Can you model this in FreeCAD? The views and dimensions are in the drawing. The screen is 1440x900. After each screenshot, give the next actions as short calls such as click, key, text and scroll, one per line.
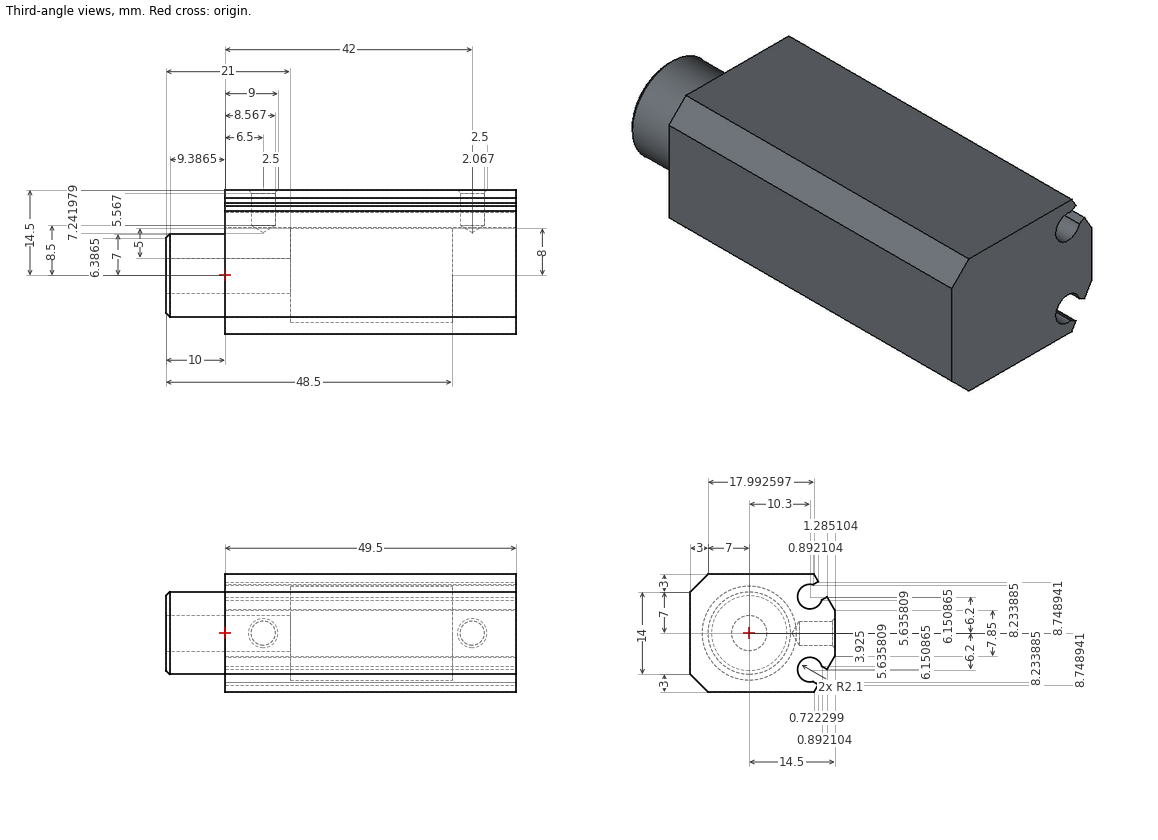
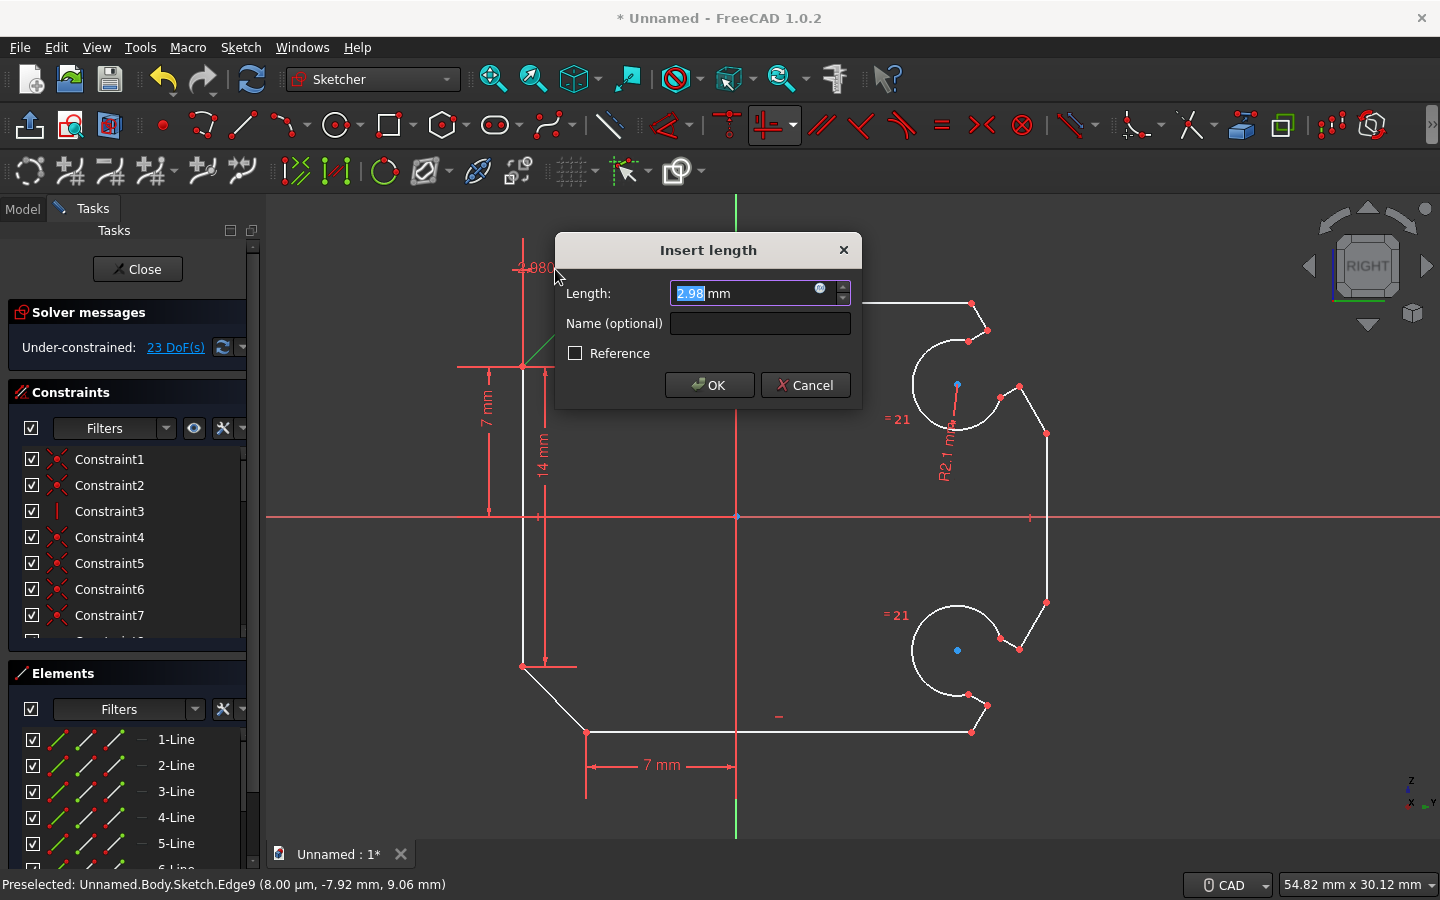
text(3)
key(Return)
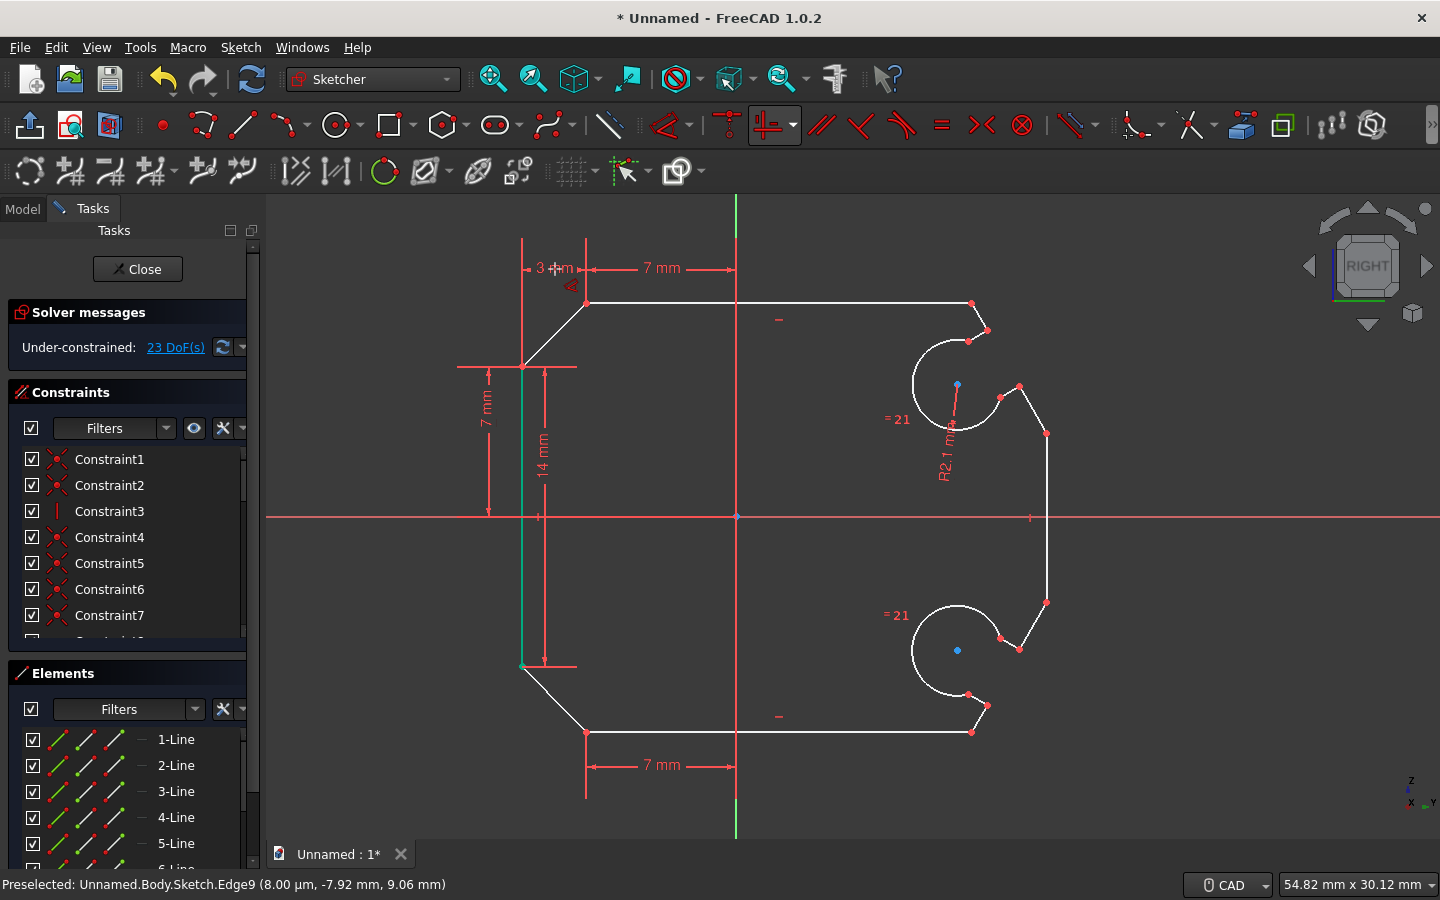
click(567, 322)
click(488, 335)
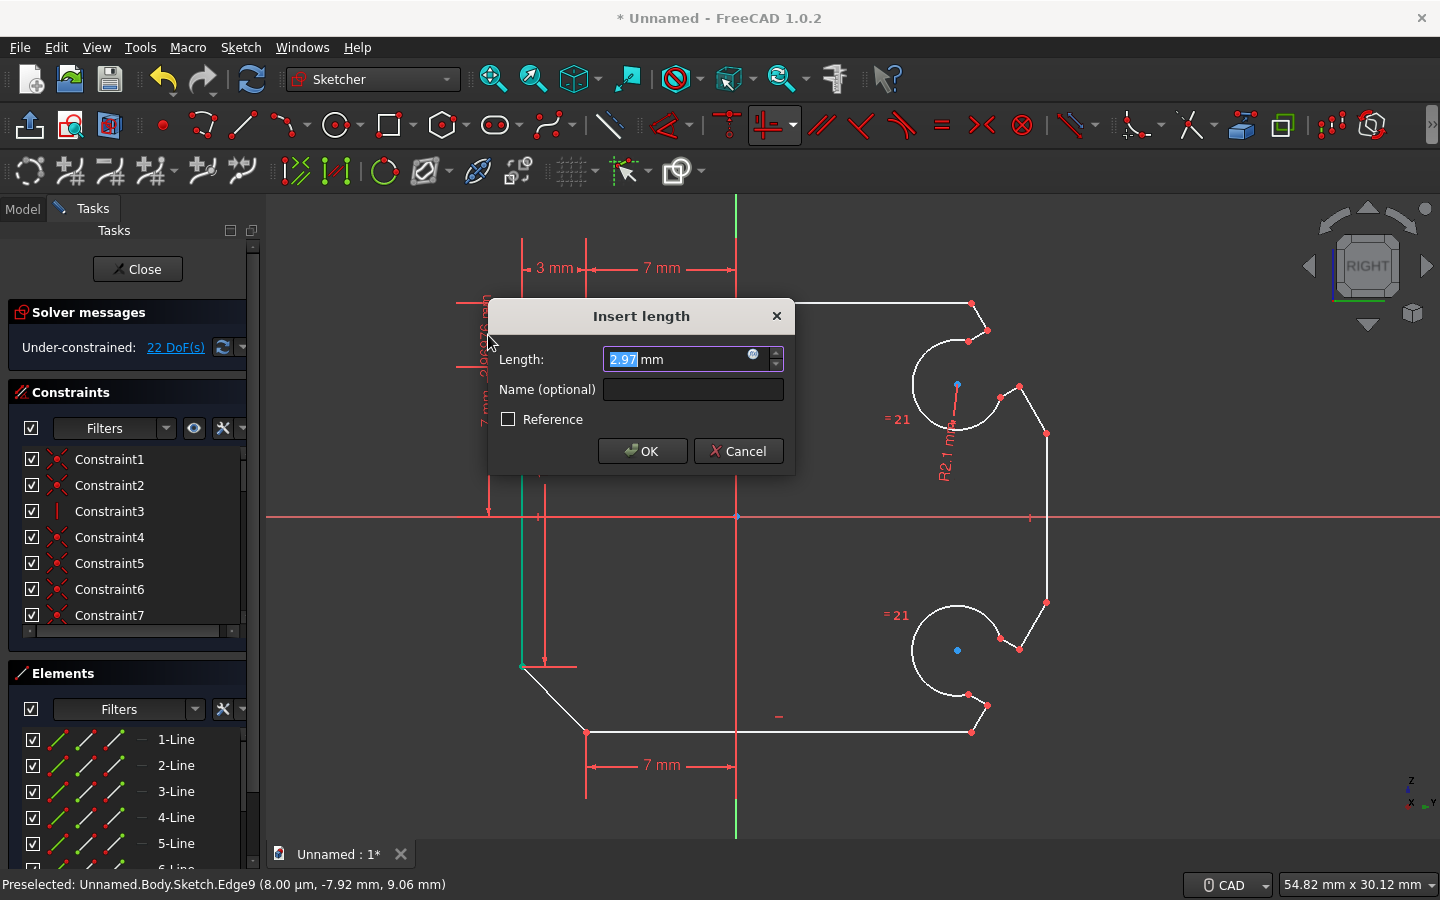
text(3)
key(Return)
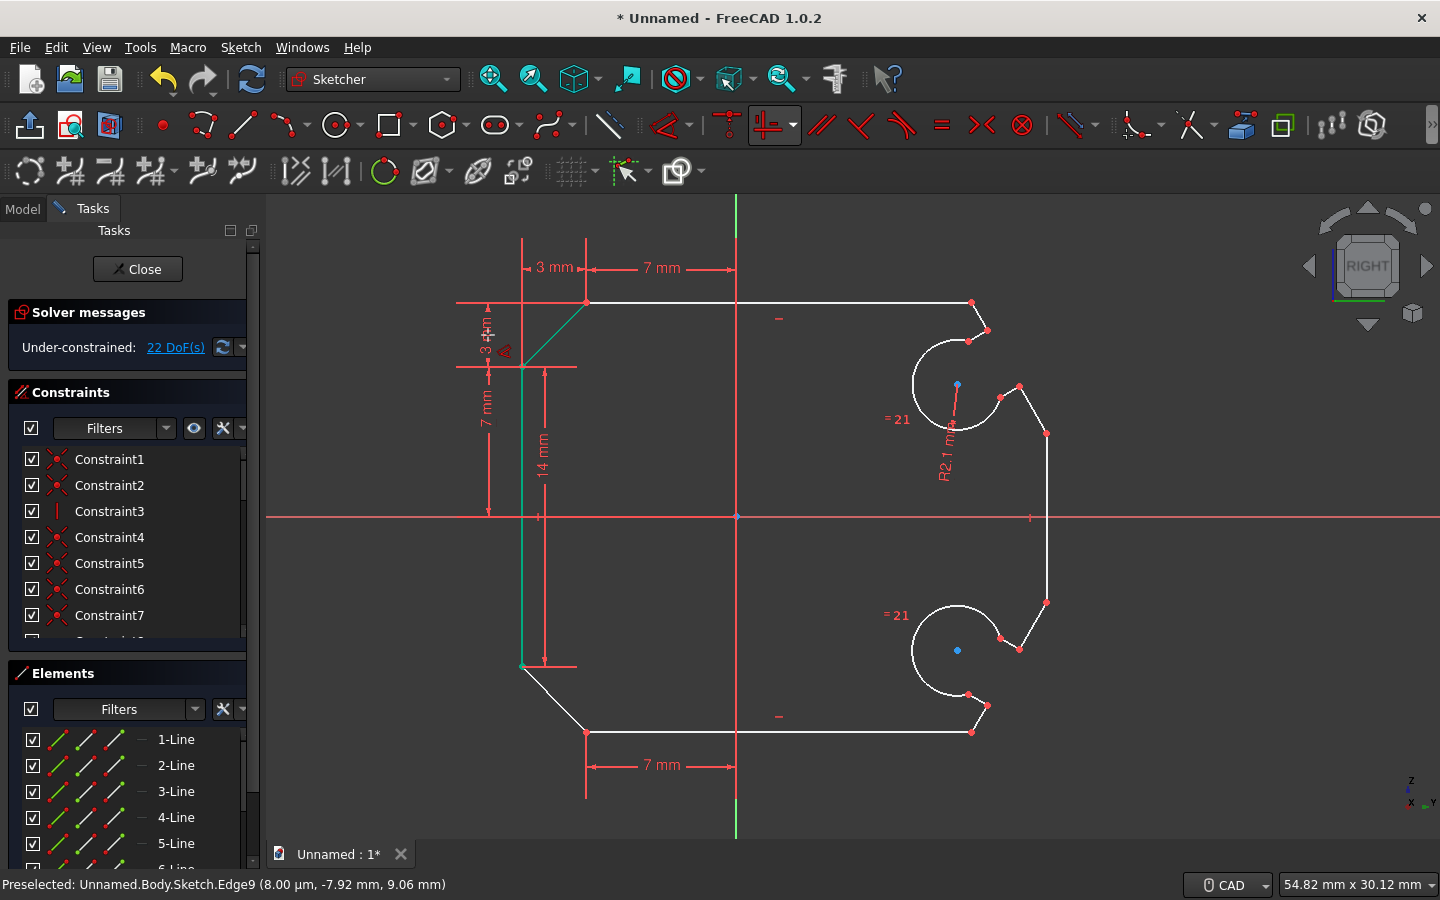
click(542, 686)
click(488, 700)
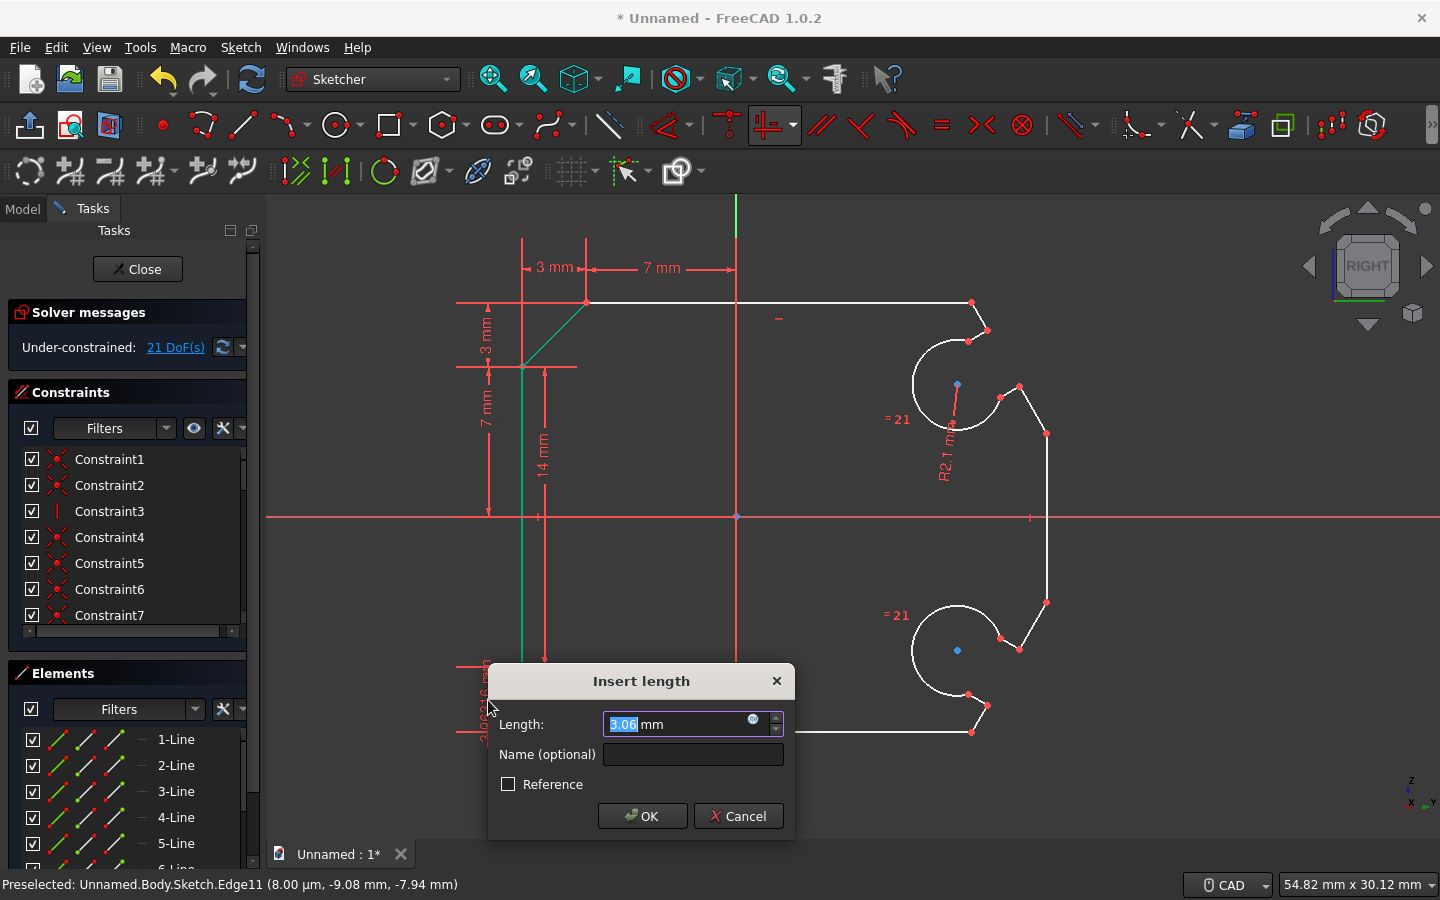
text(3)
key(Return)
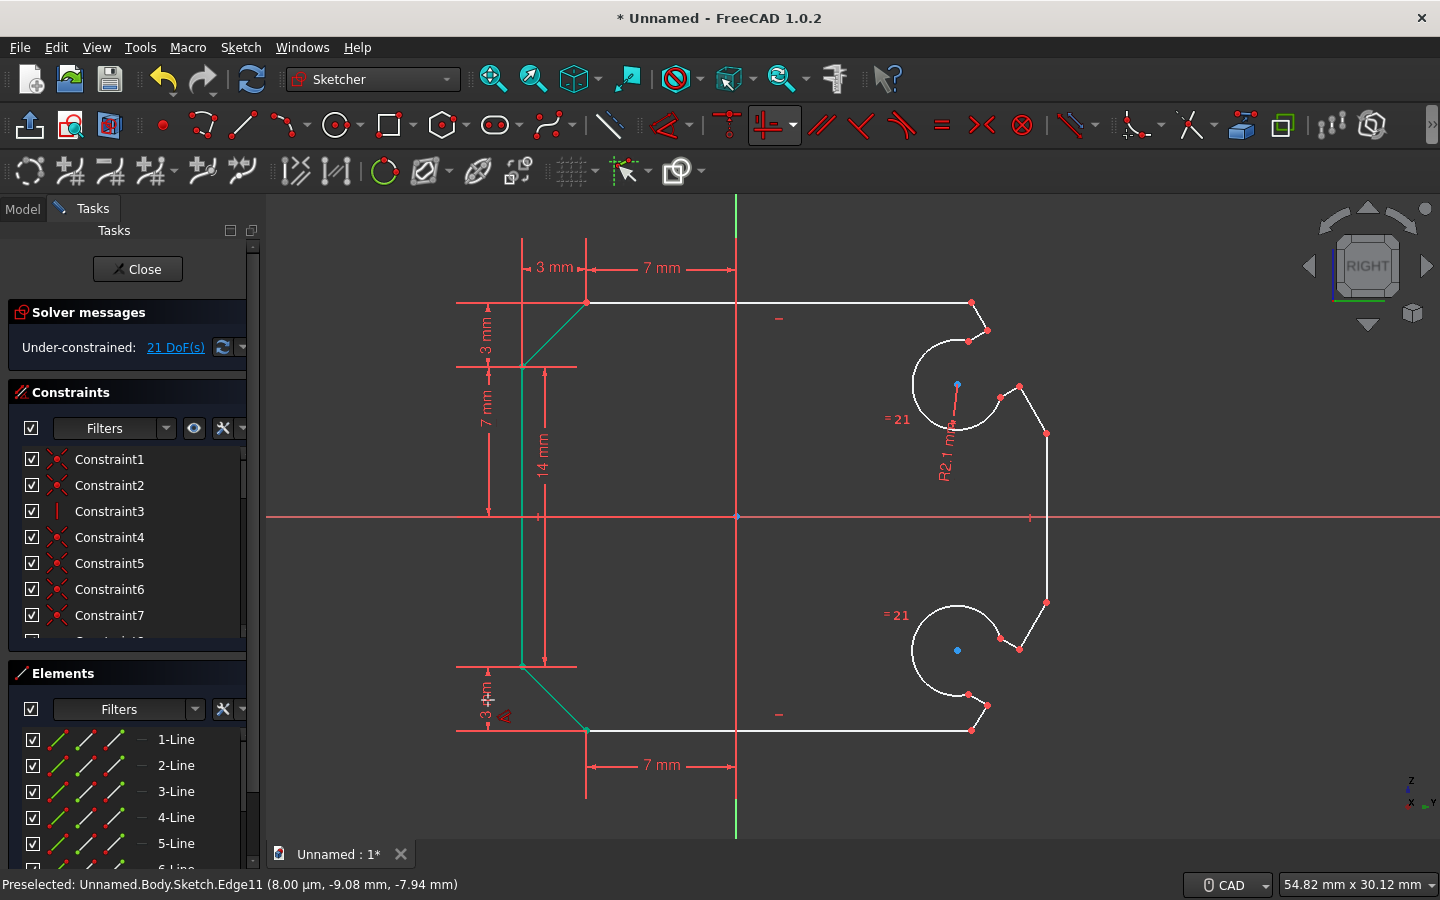
click(1047, 552)
click(1081, 479)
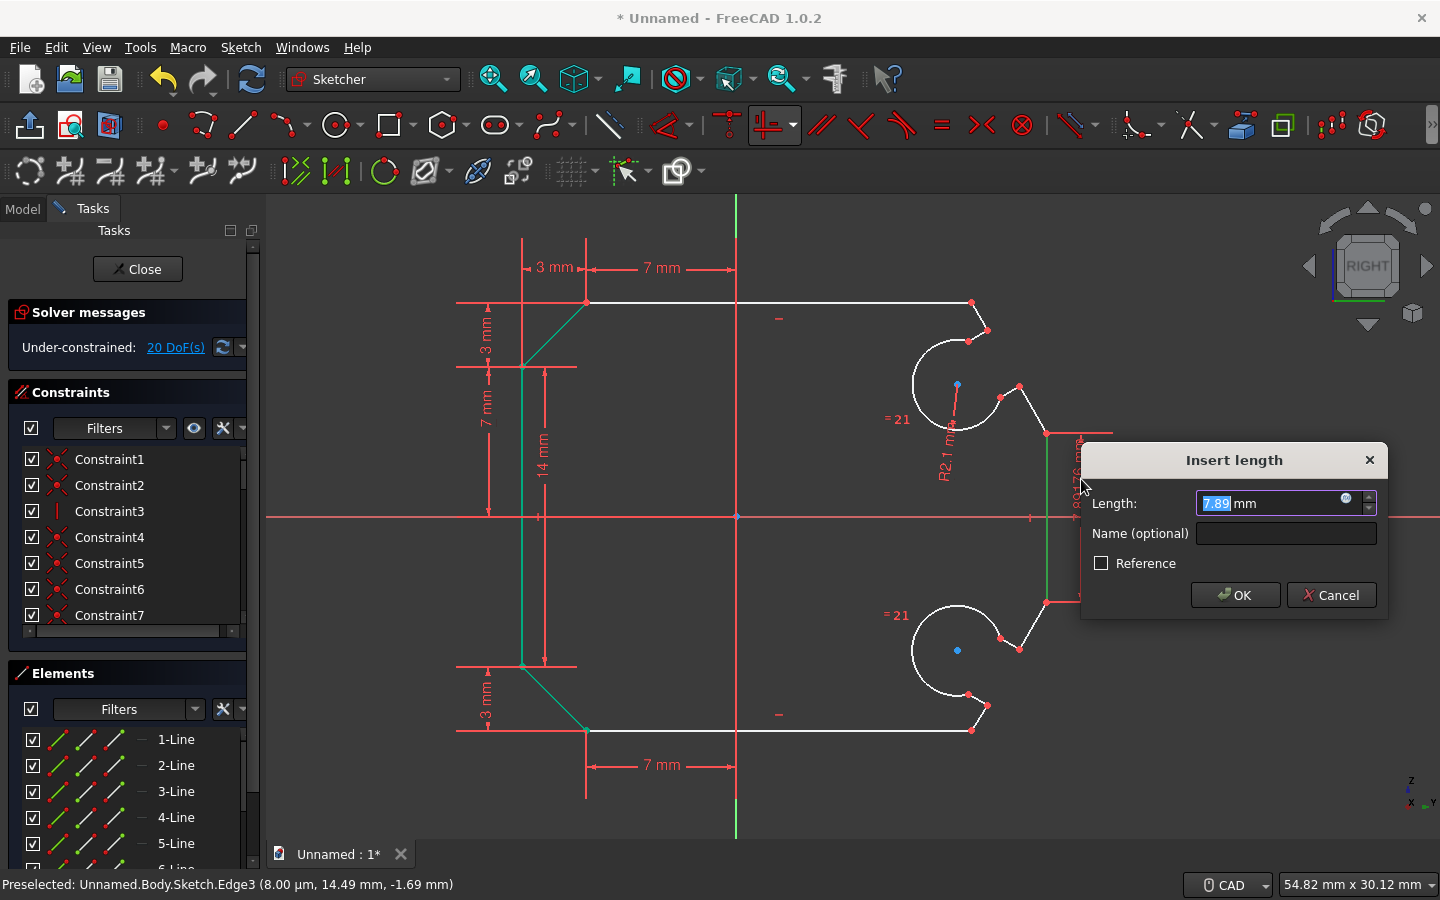
text(7.85)
key(Return)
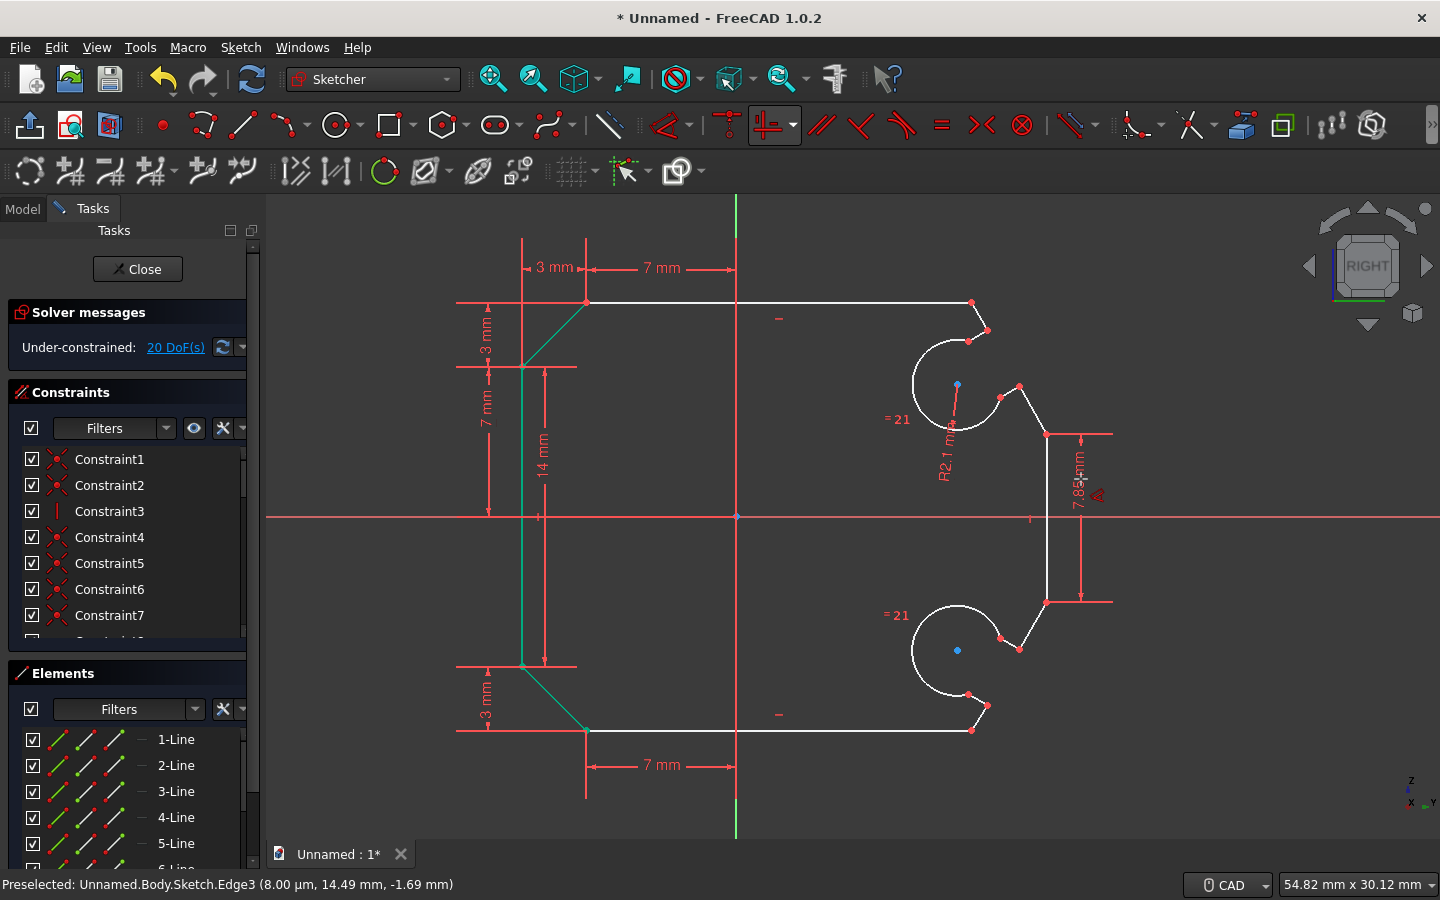
click(957, 385)
click(991, 481)